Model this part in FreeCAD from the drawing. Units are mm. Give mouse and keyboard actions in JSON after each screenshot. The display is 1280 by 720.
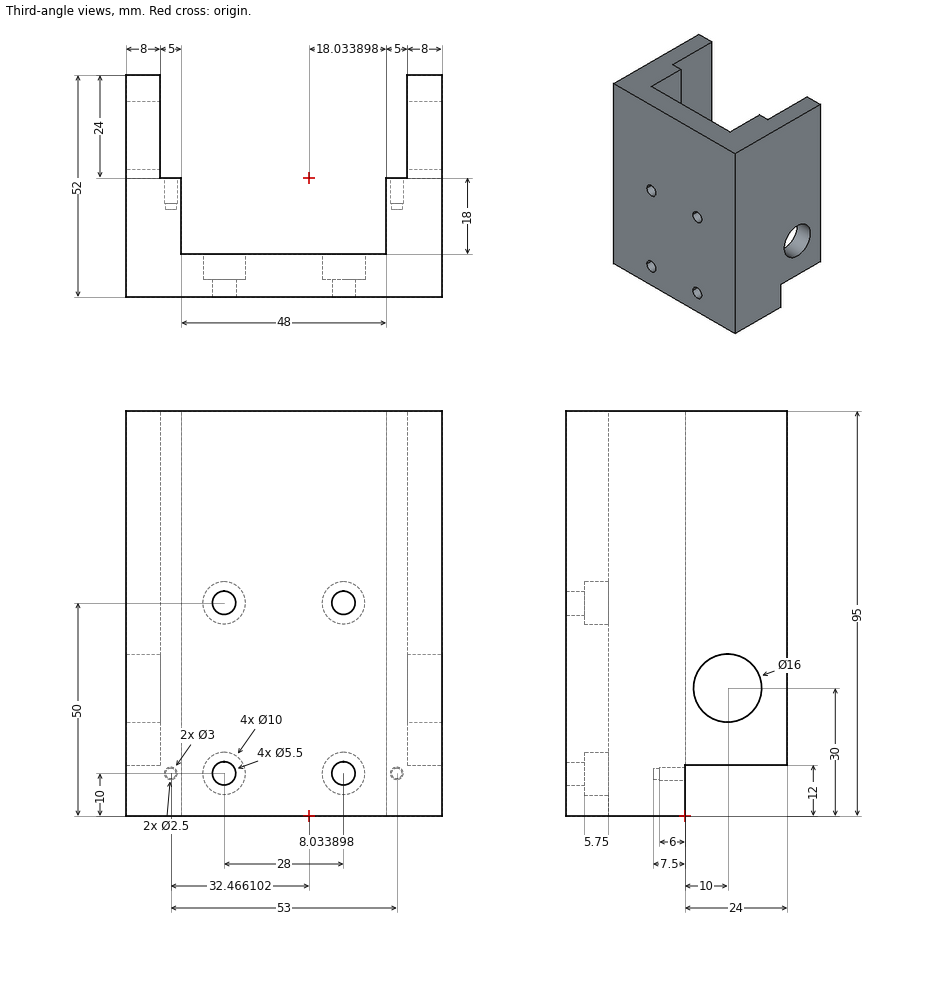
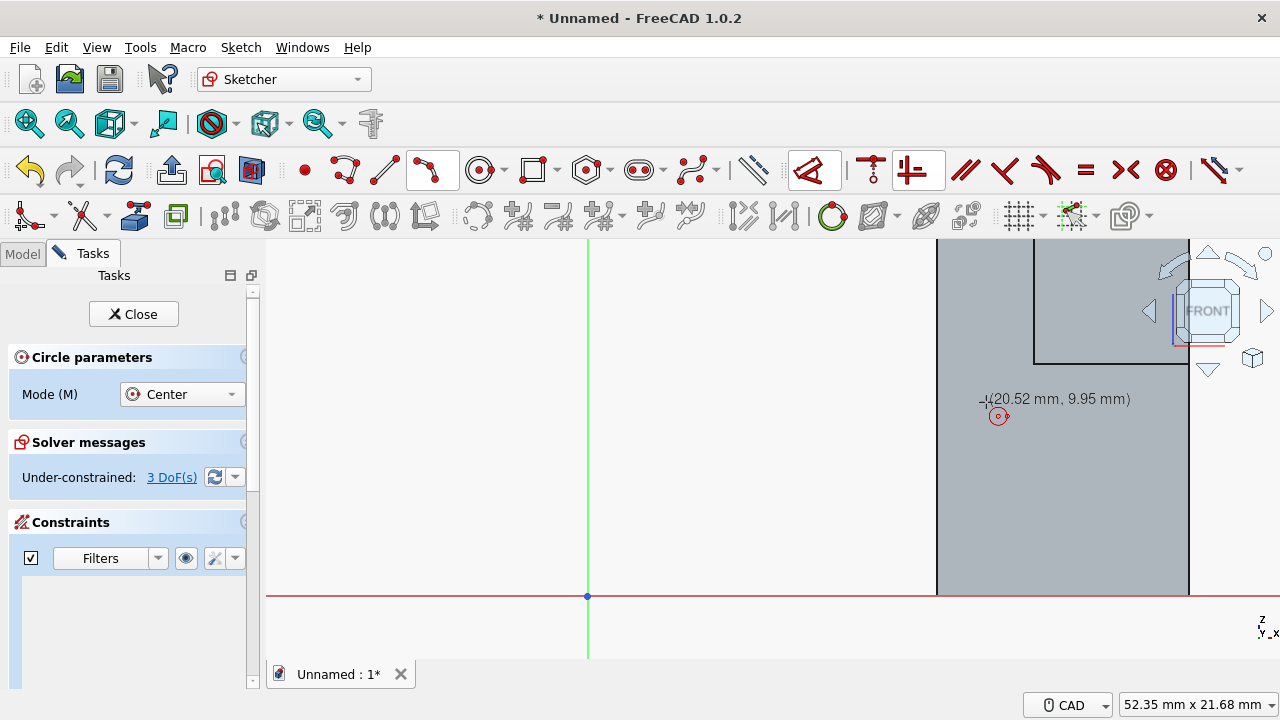
{"action": "left_click", "coordinate": [986, 402]}
{"action": "left_click", "coordinate": [1003, 385]}
{"action": "key", "text": "Escape"}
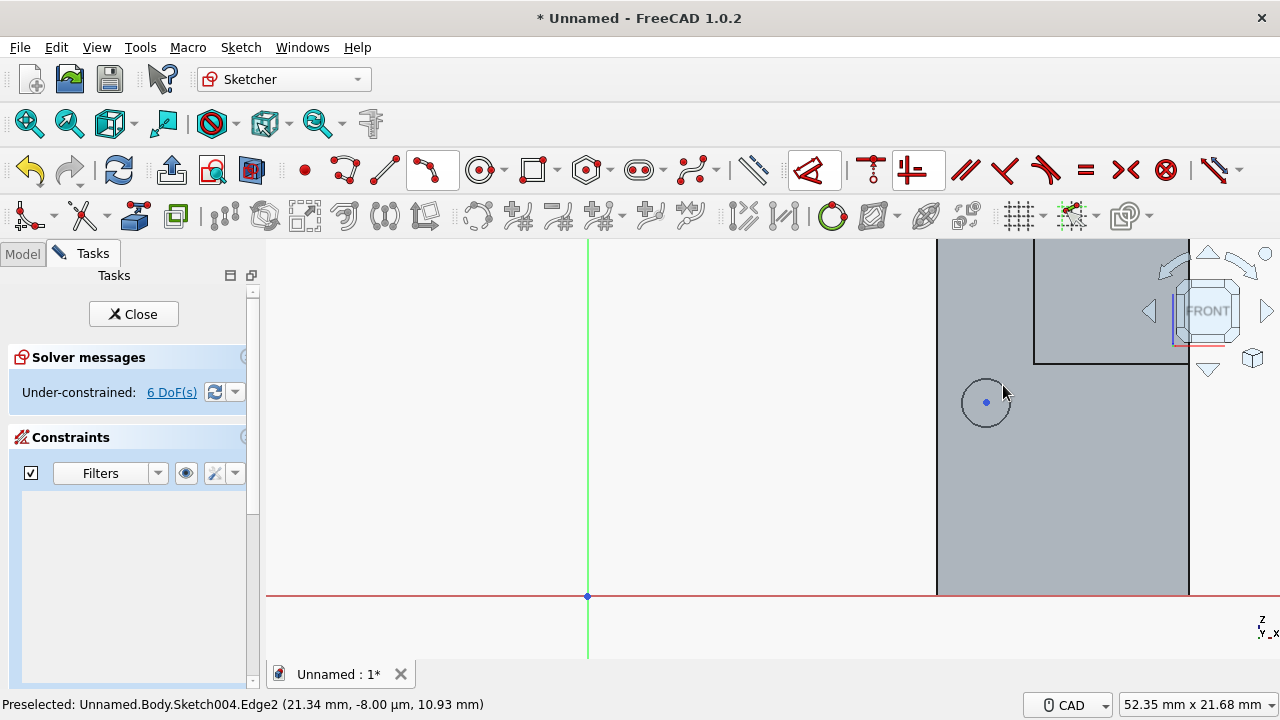
{"action": "scroll", "coordinate": [987, 403], "scroll_direction": "down", "scroll_amount": 3}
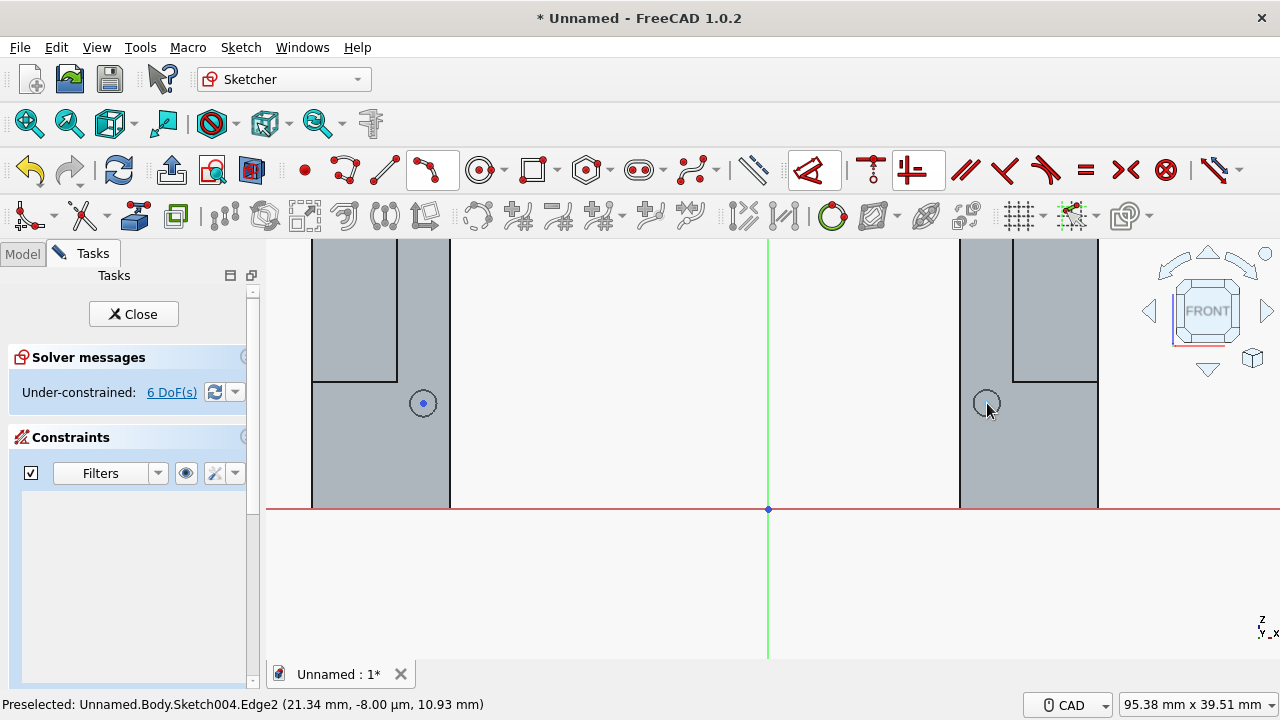
{"action": "left_click", "coordinate": [433, 394]}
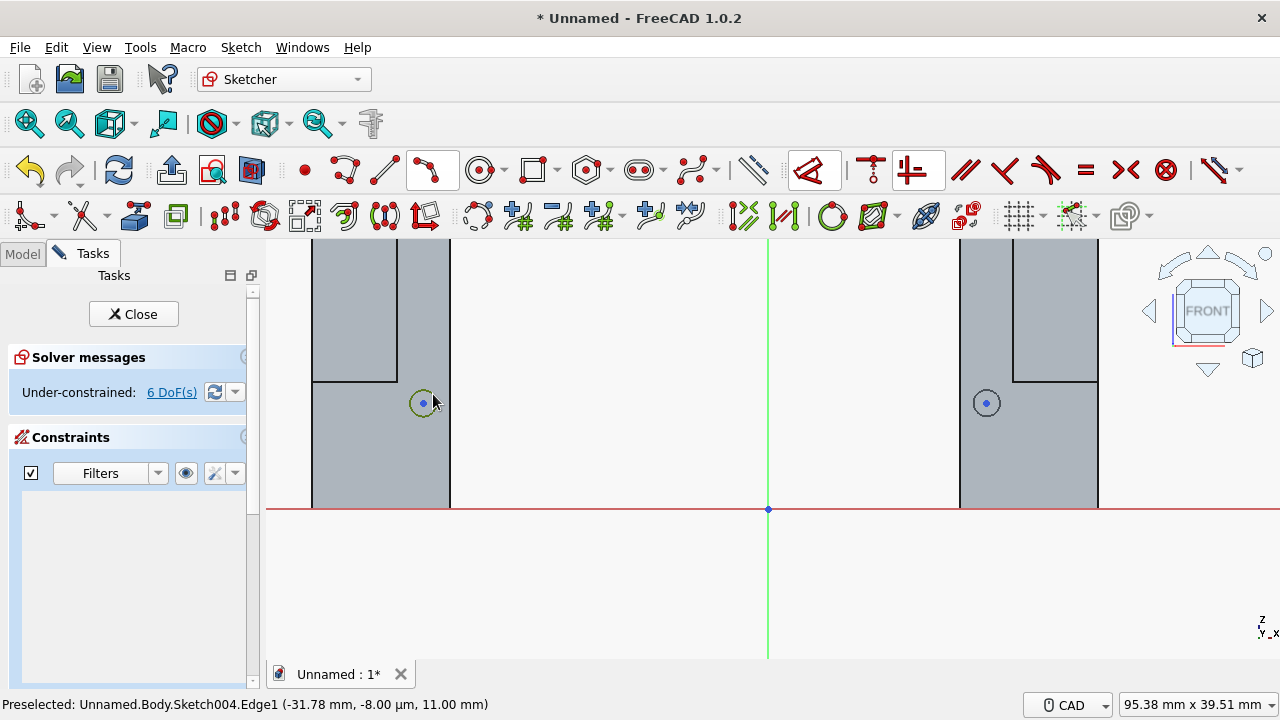
{"action": "left_click", "coordinate": [996, 394]}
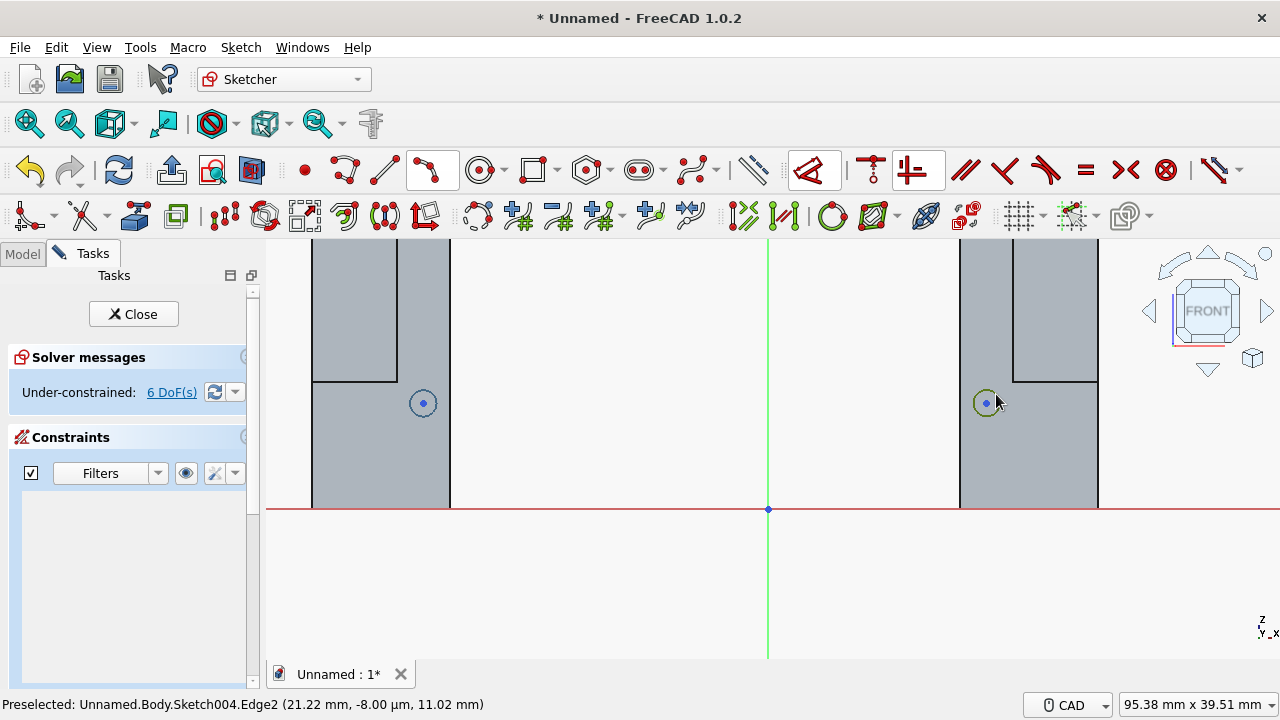
{"action": "left_click", "coordinate": [1086, 170]}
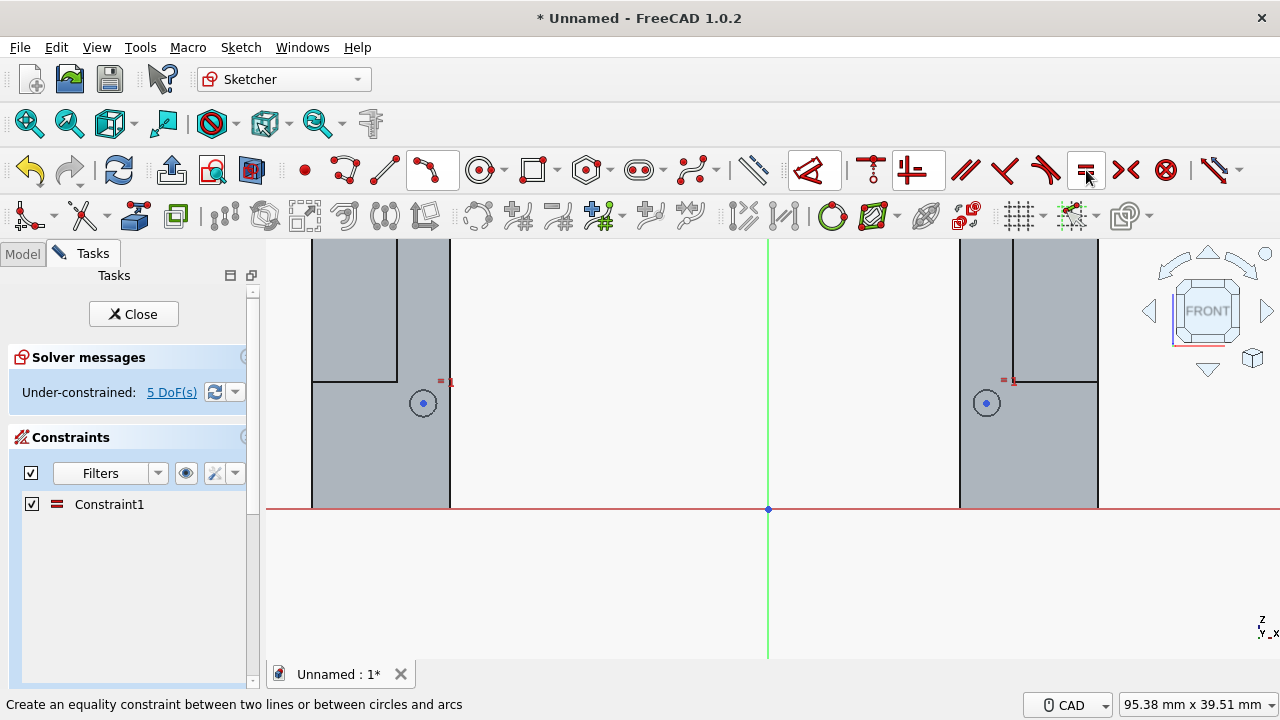
{"action": "left_click", "coordinate": [423, 403]}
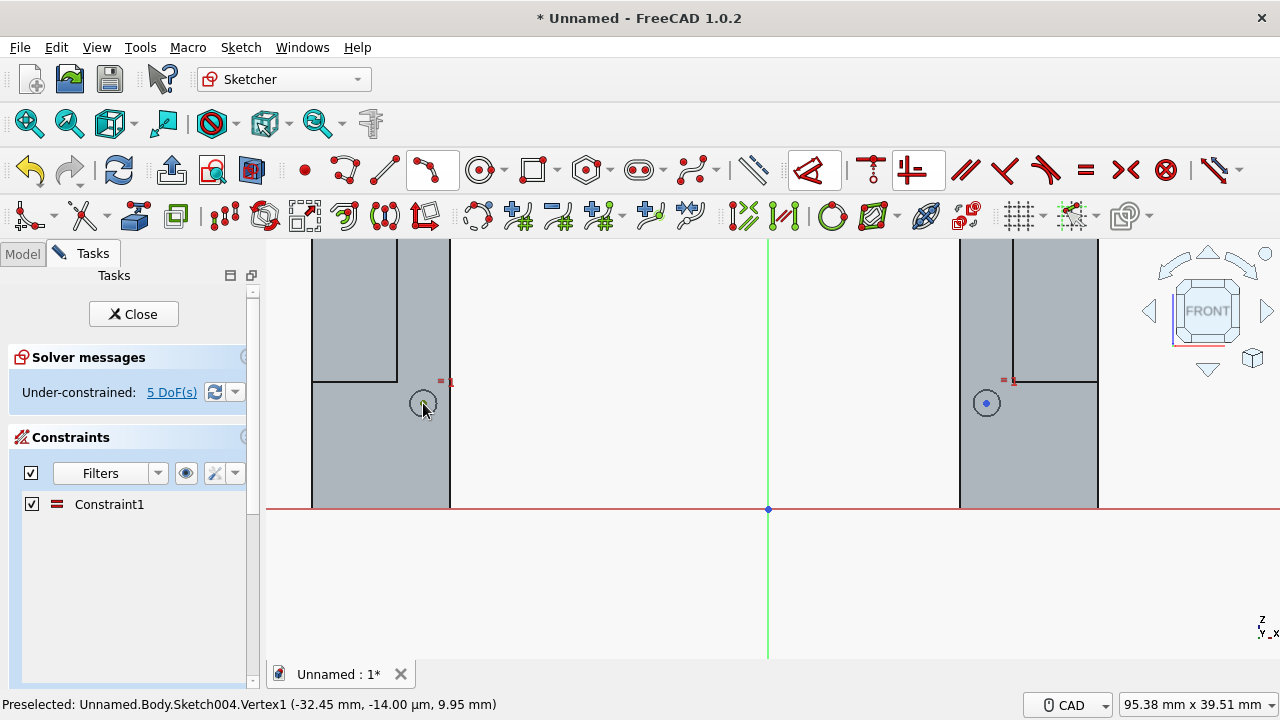
{"action": "left_click", "coordinate": [987, 403]}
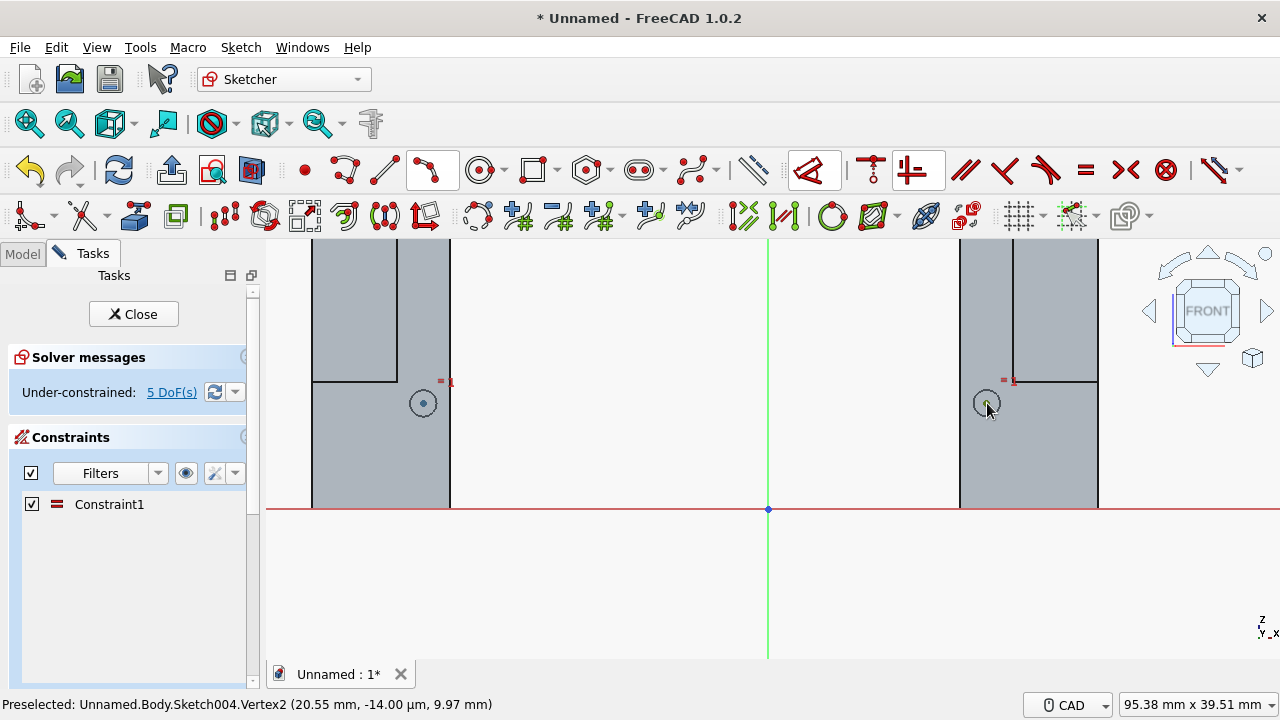
{"action": "key", "text": "h"}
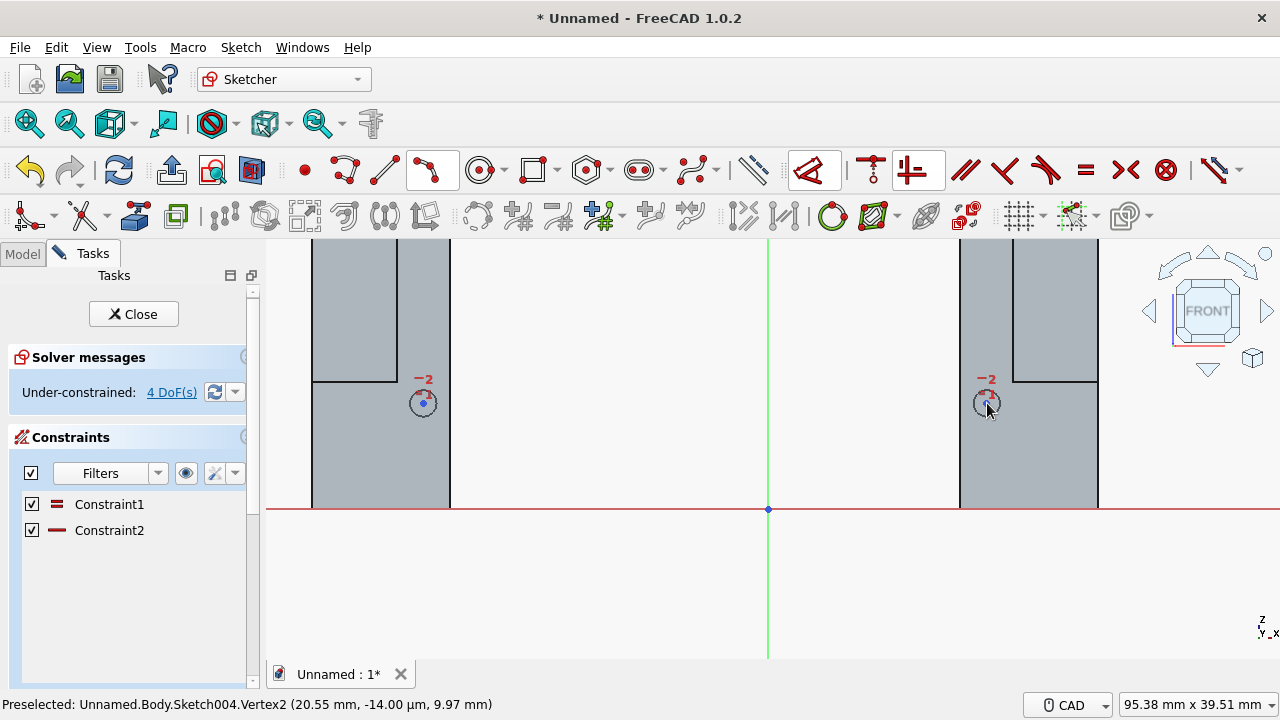
{"action": "scroll", "coordinate": [433, 394], "scroll_direction": "up", "scroll_amount": 3}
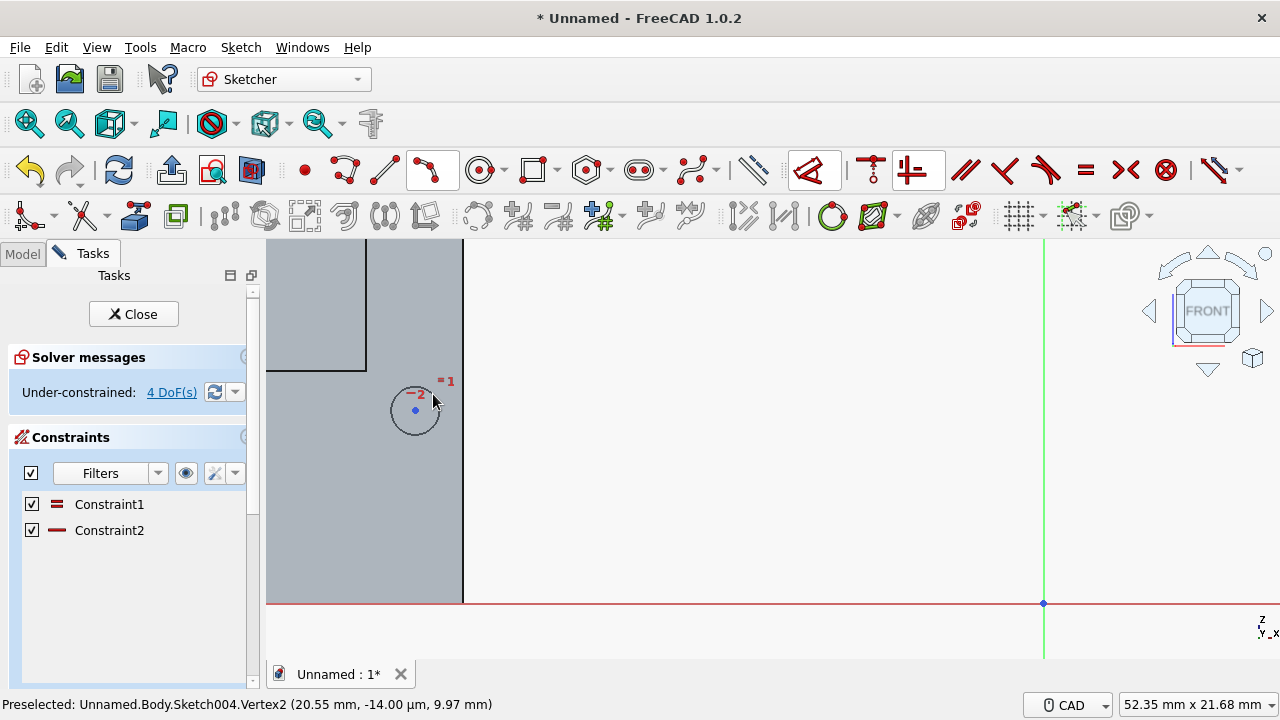
{"action": "left_click", "coordinate": [432, 394]}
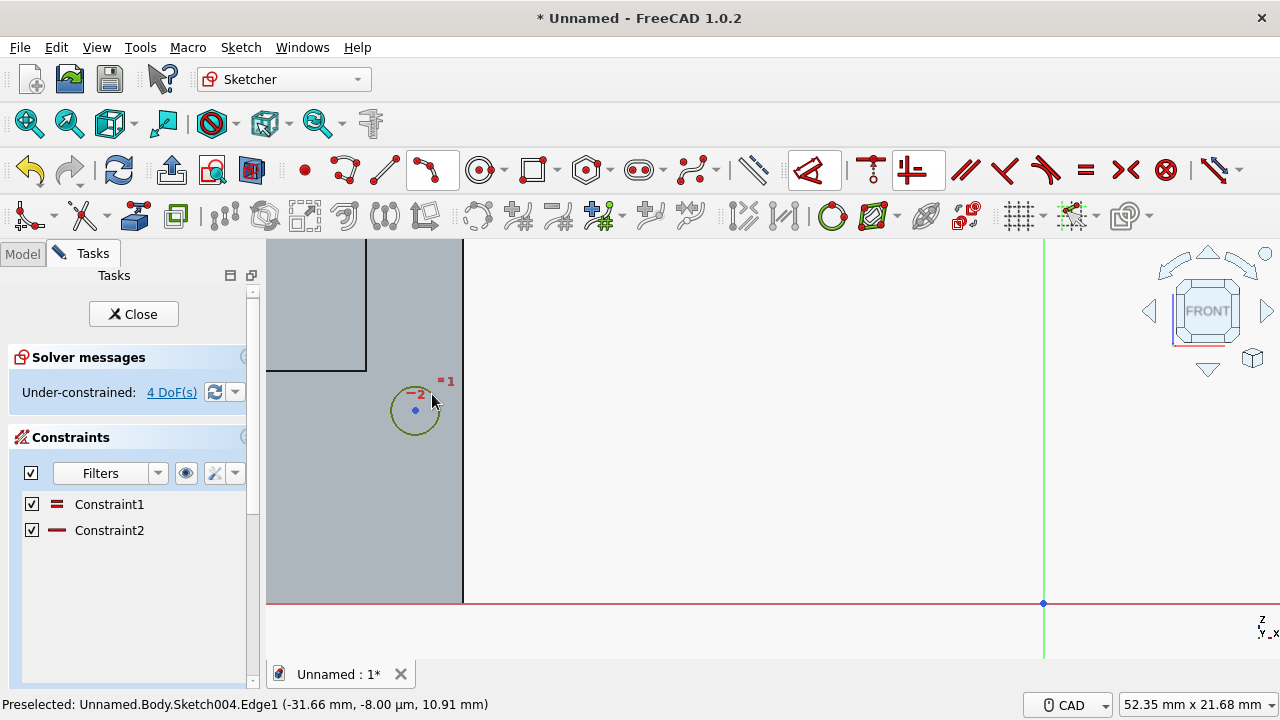
{"action": "key", "text": "k o"}